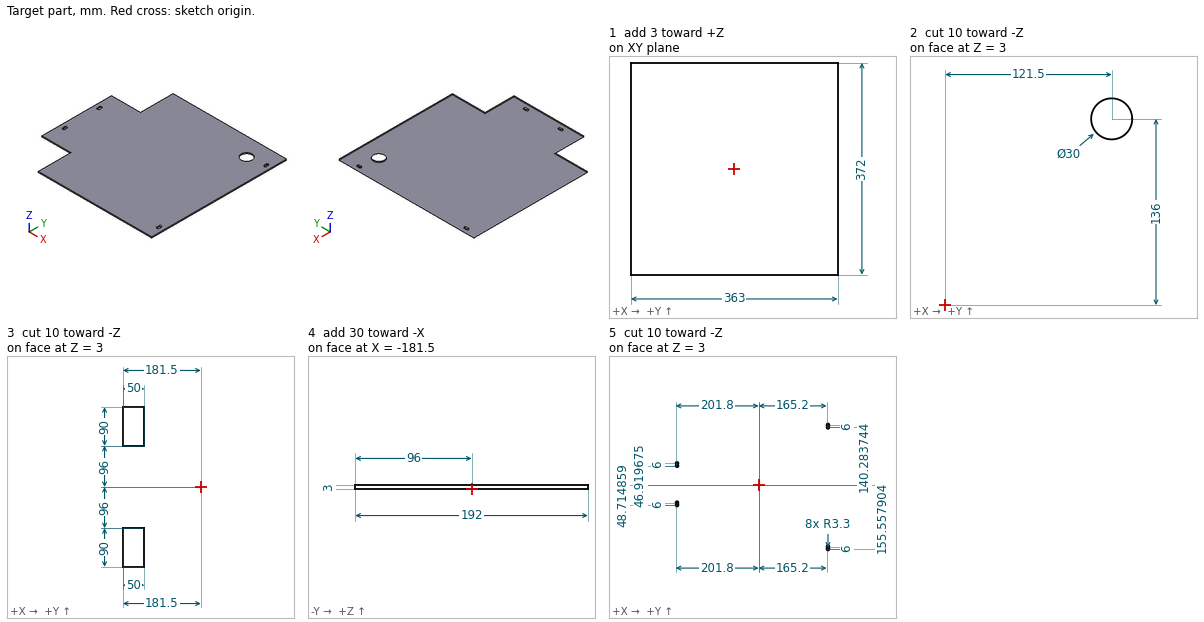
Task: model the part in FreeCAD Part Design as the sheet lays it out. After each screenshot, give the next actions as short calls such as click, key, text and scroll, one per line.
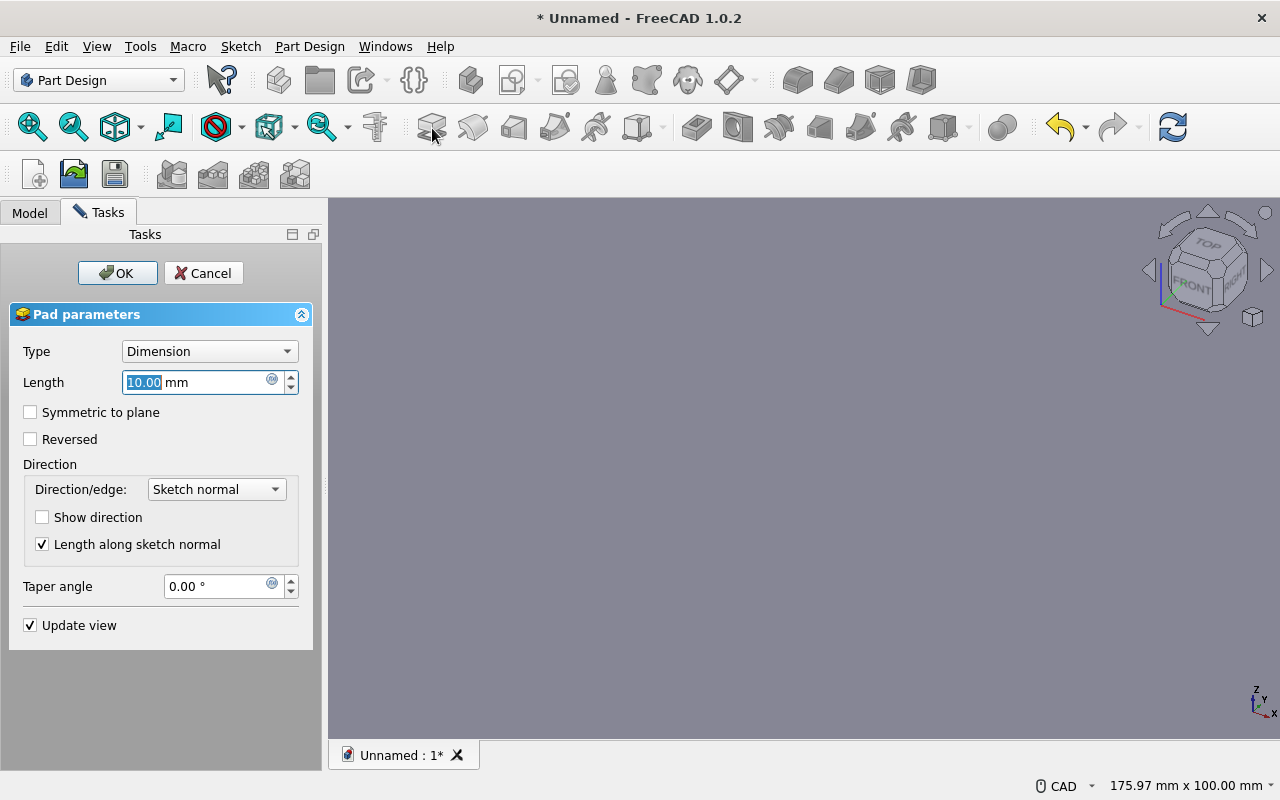
text(3)
key(Tab)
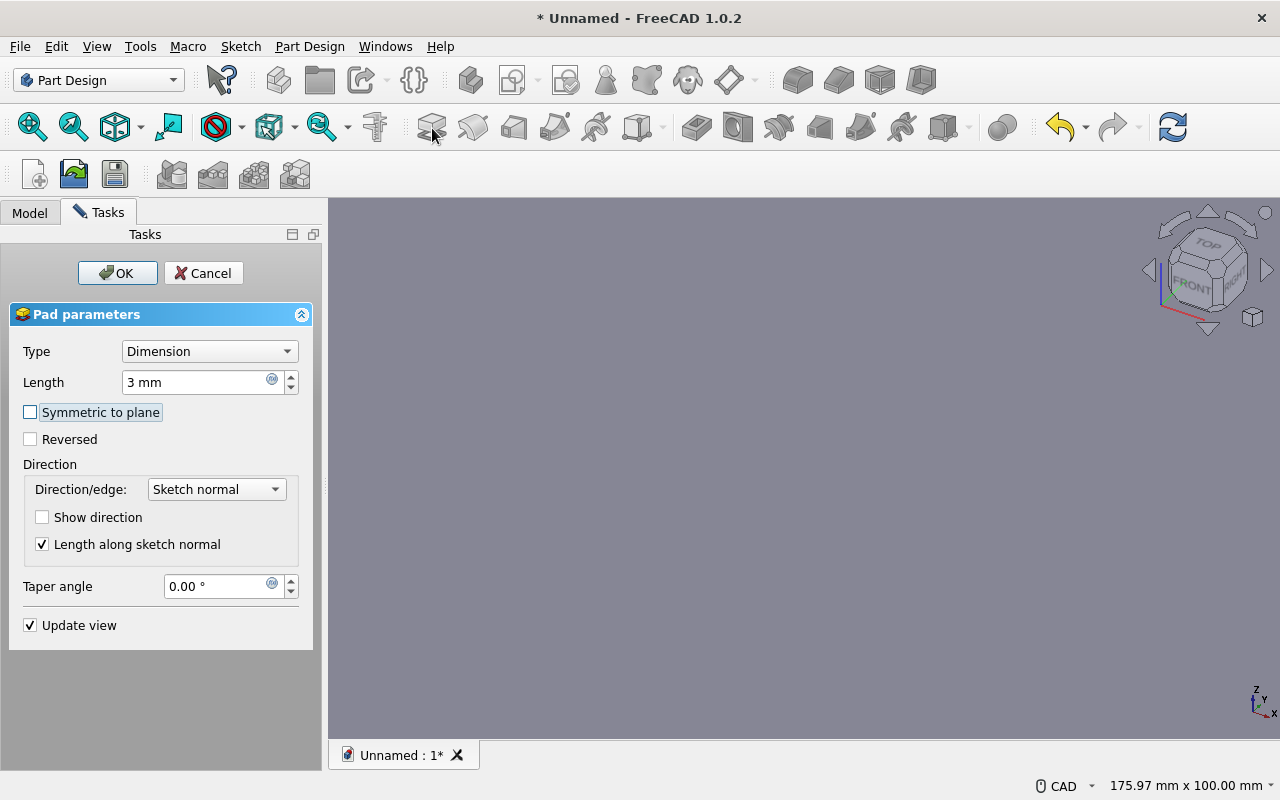
click(118, 273)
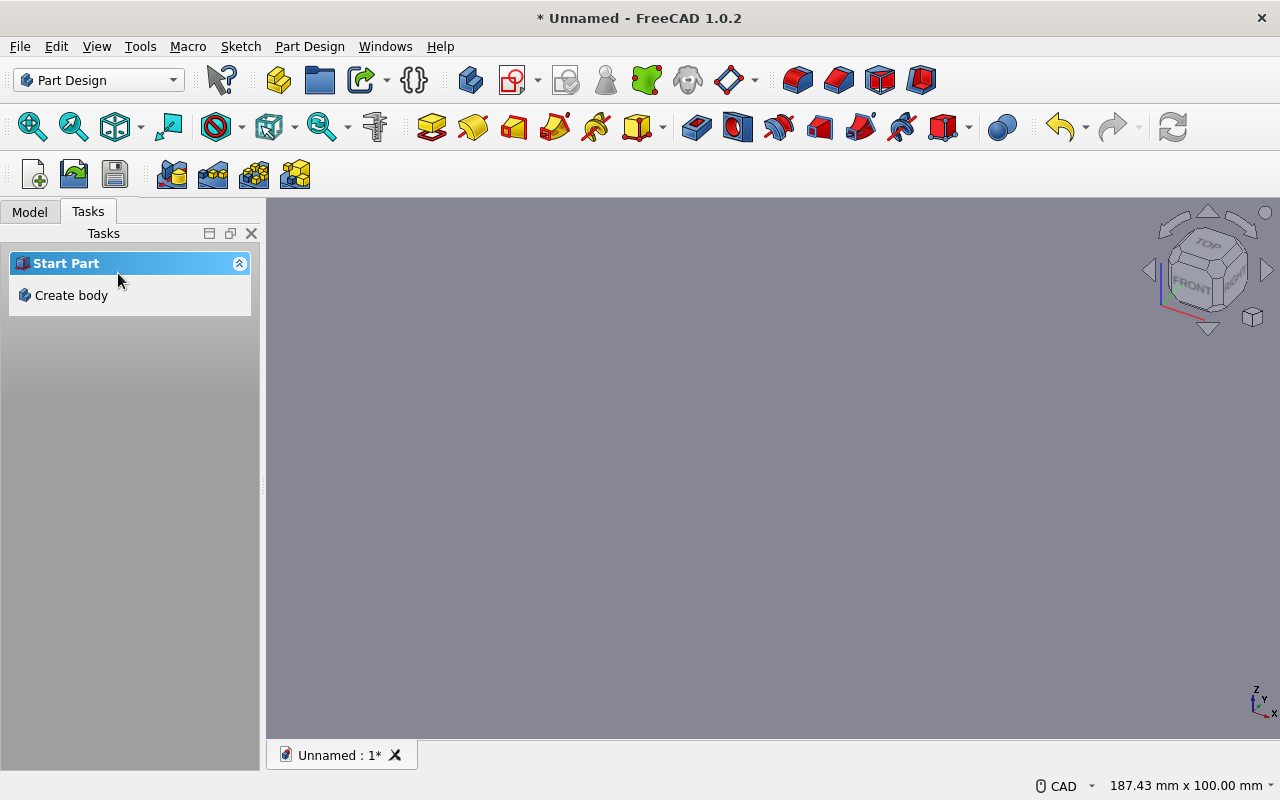
key(v)
key(f)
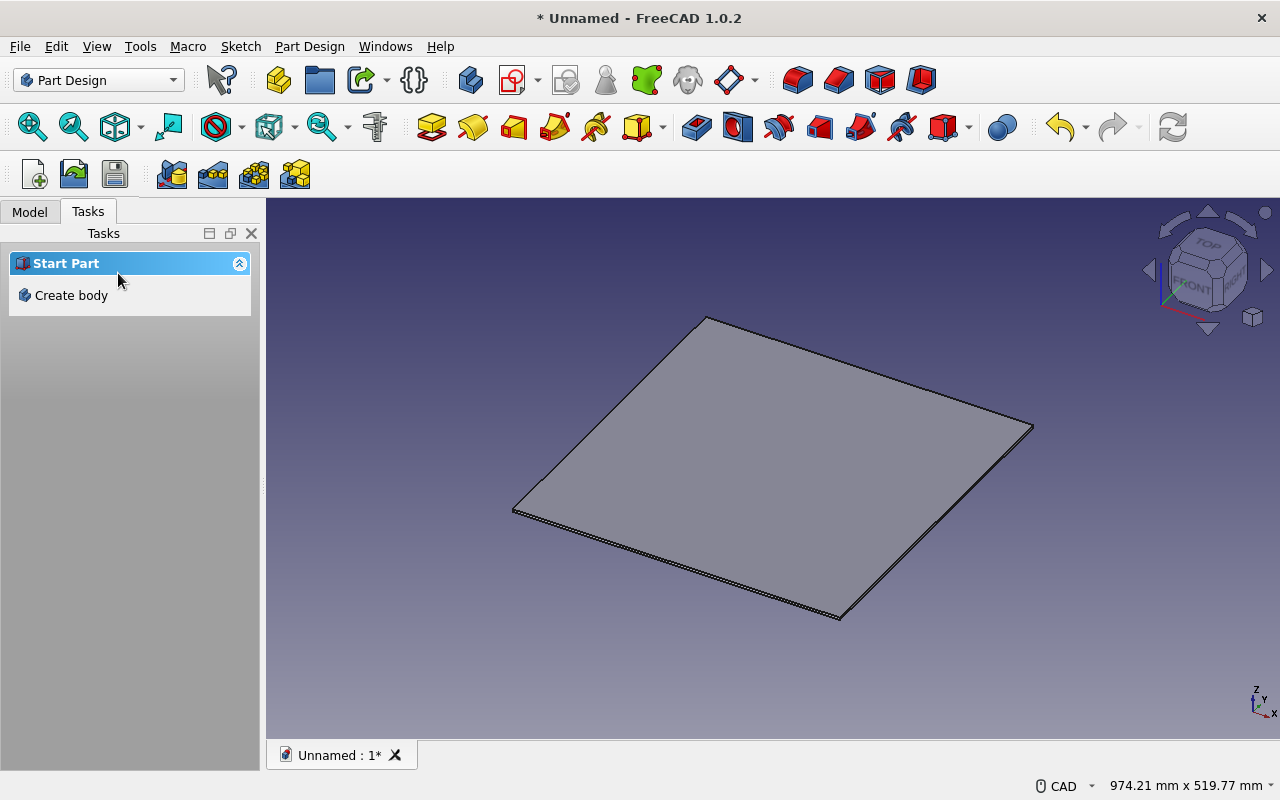
click(773, 466)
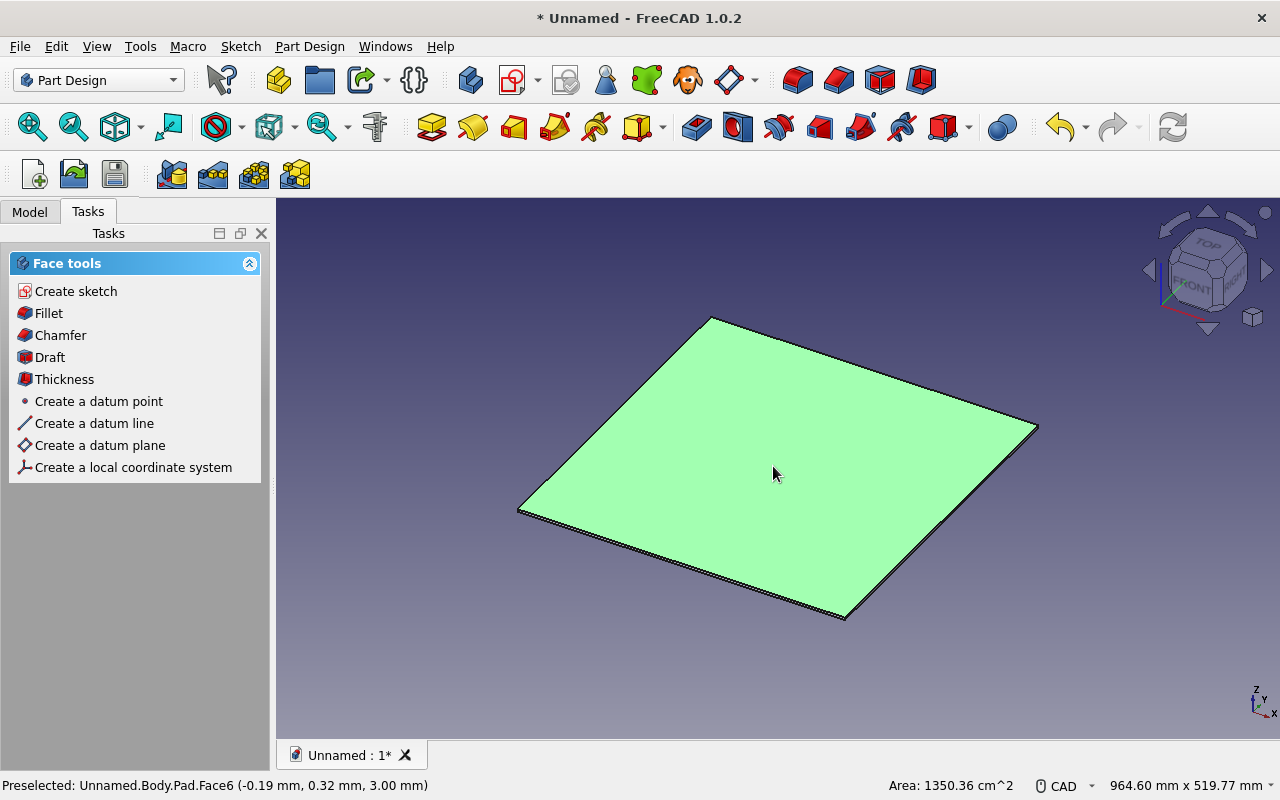
click(512, 80)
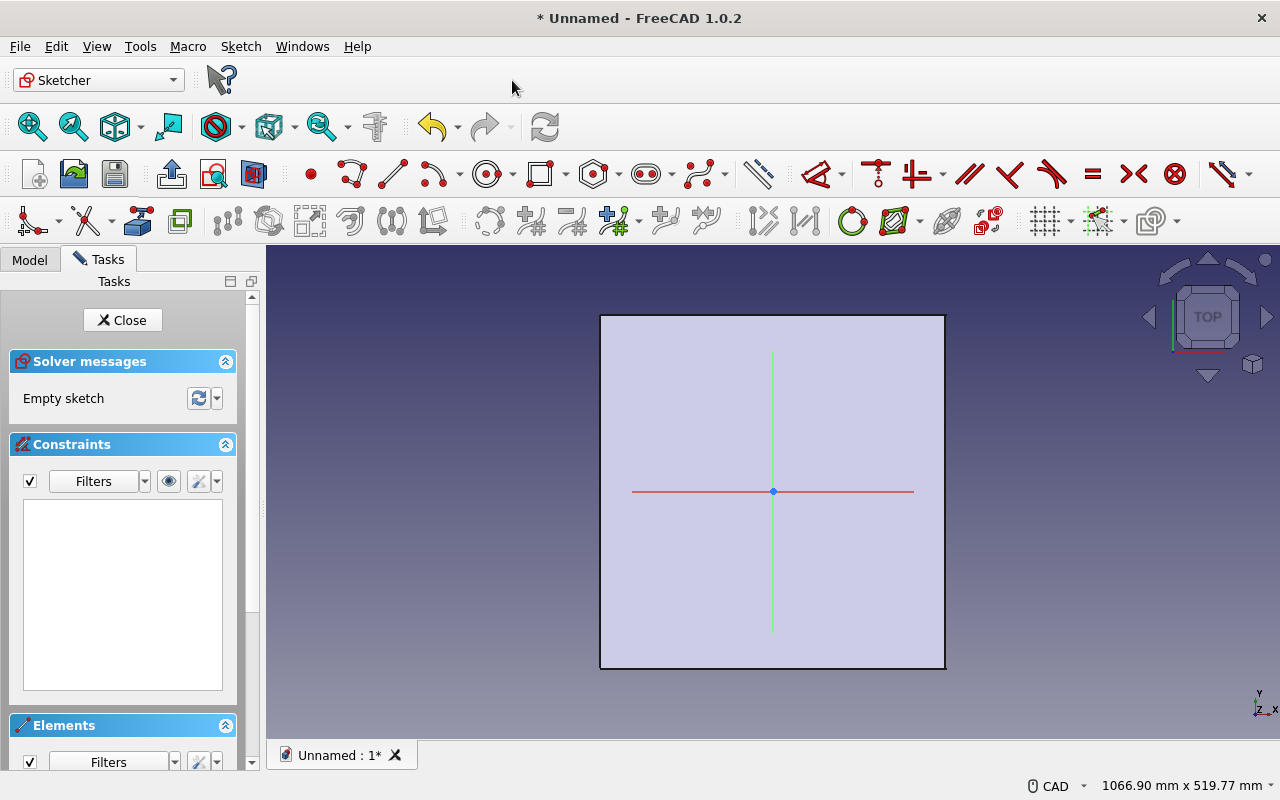
scroll(907, 350, up, 12)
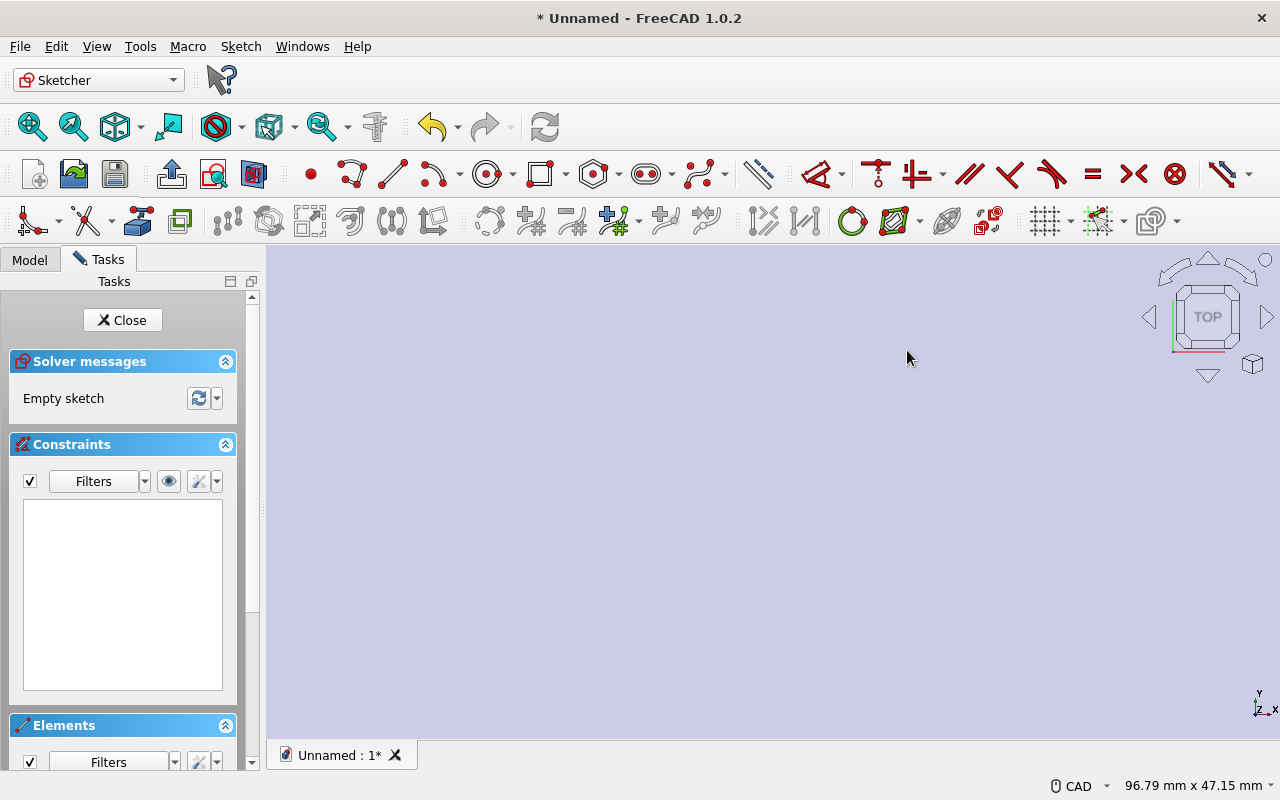
key(g)
key(c)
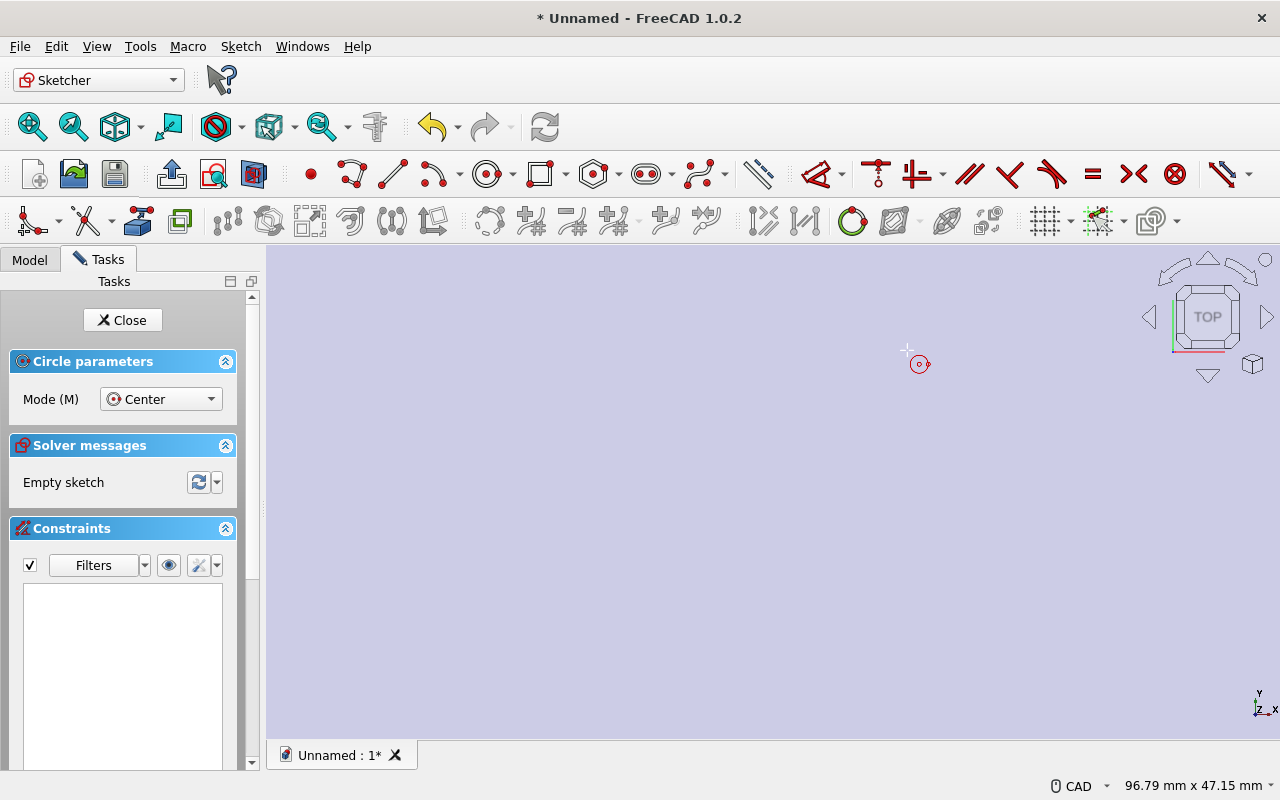
click(696, 488)
move(808, 377)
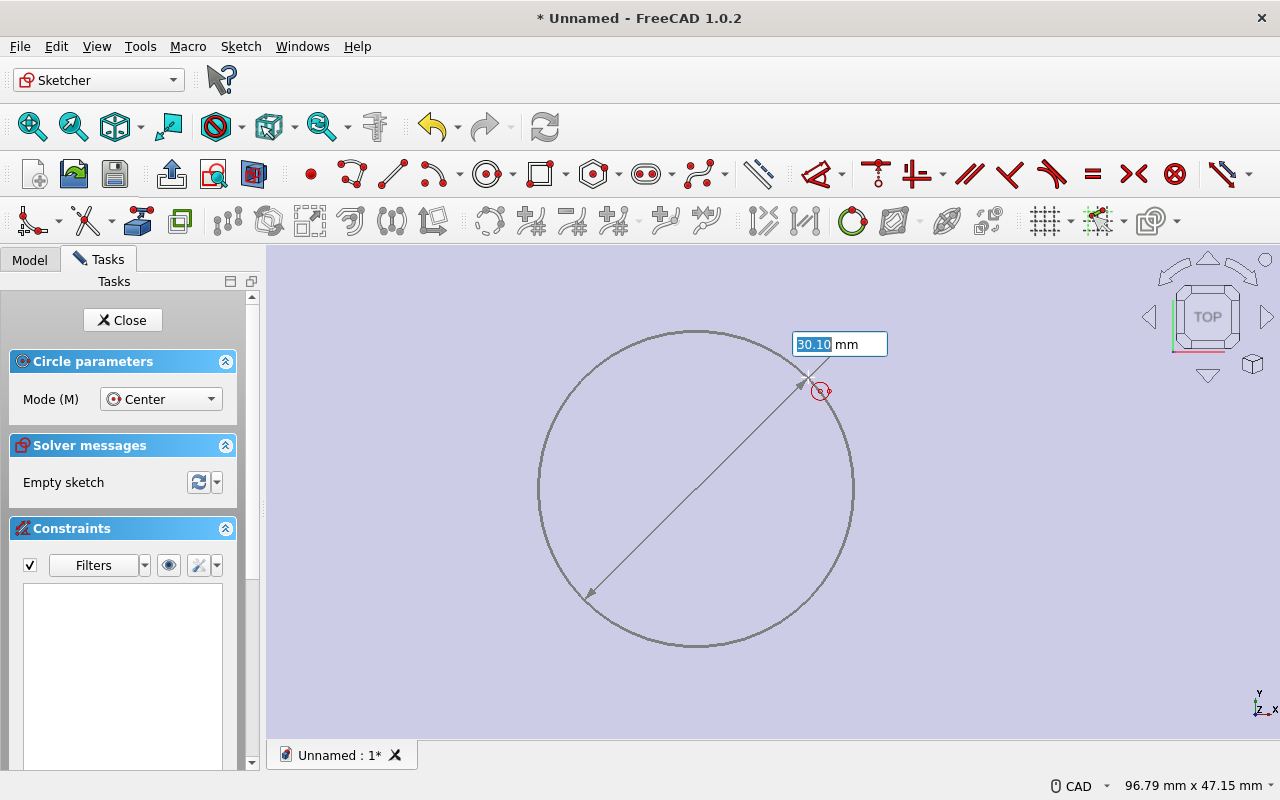
text(30)
key(Return)
key(Escape)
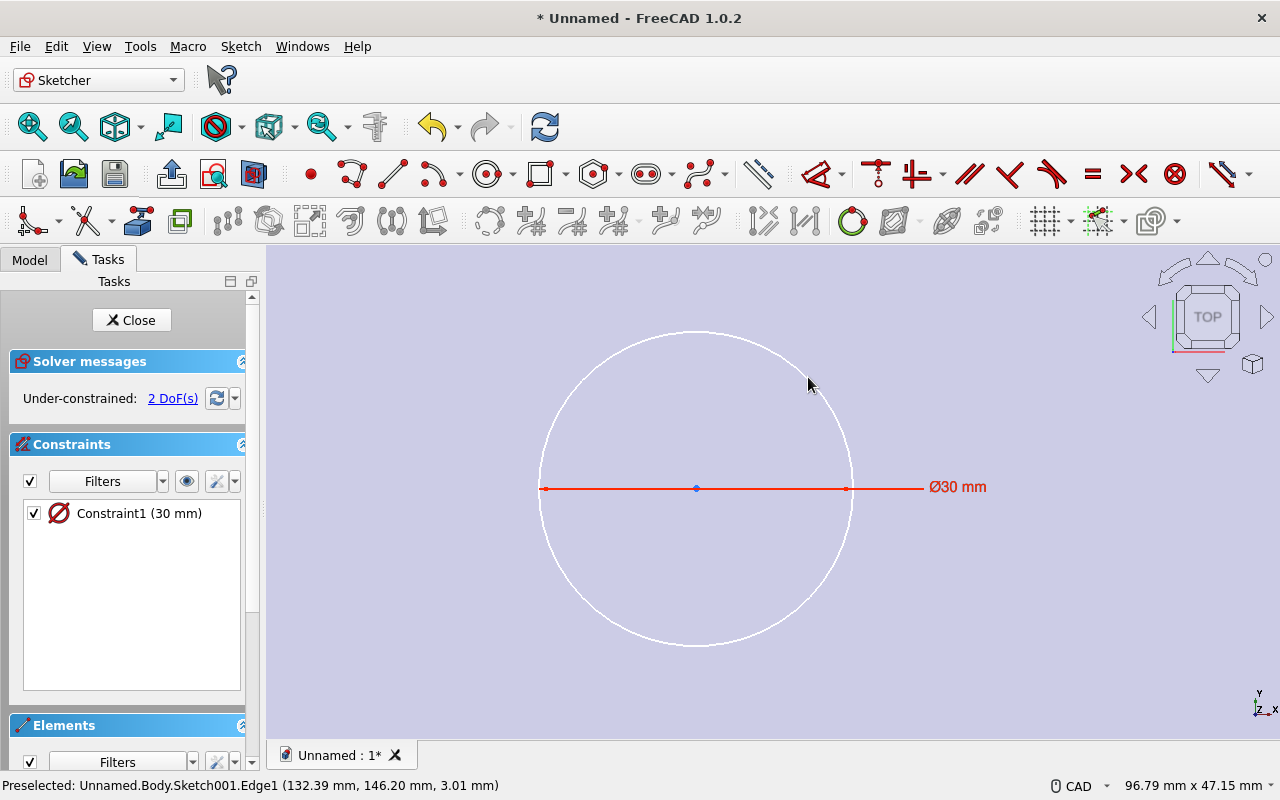
click(696, 489)